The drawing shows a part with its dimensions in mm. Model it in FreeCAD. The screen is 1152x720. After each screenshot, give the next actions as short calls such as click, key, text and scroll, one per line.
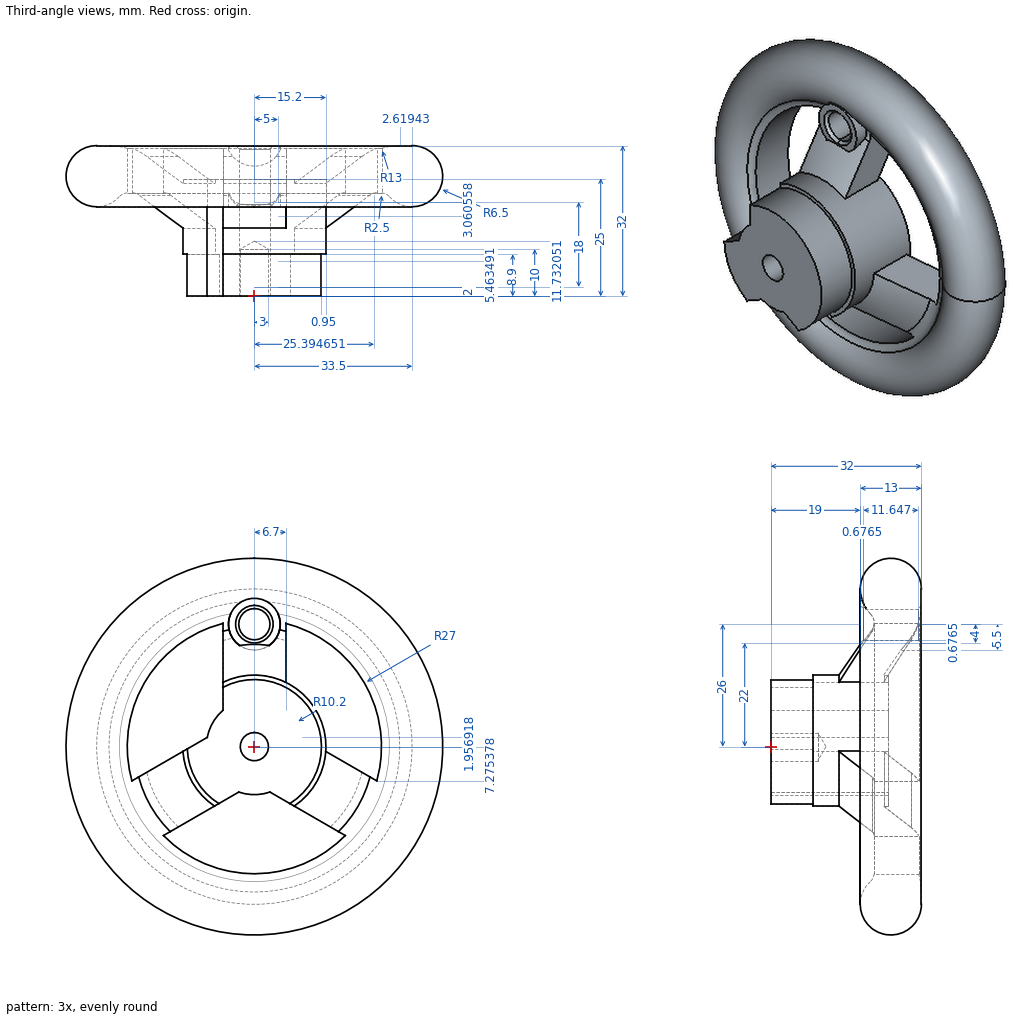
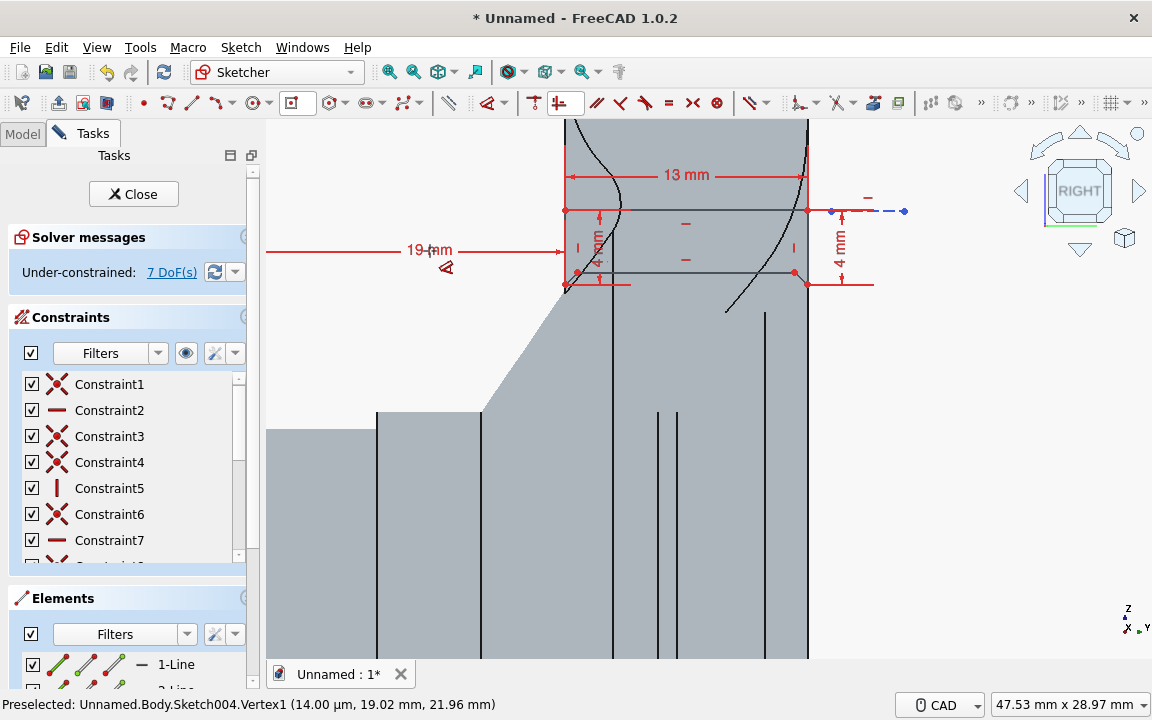
click(565, 285)
click(599, 458)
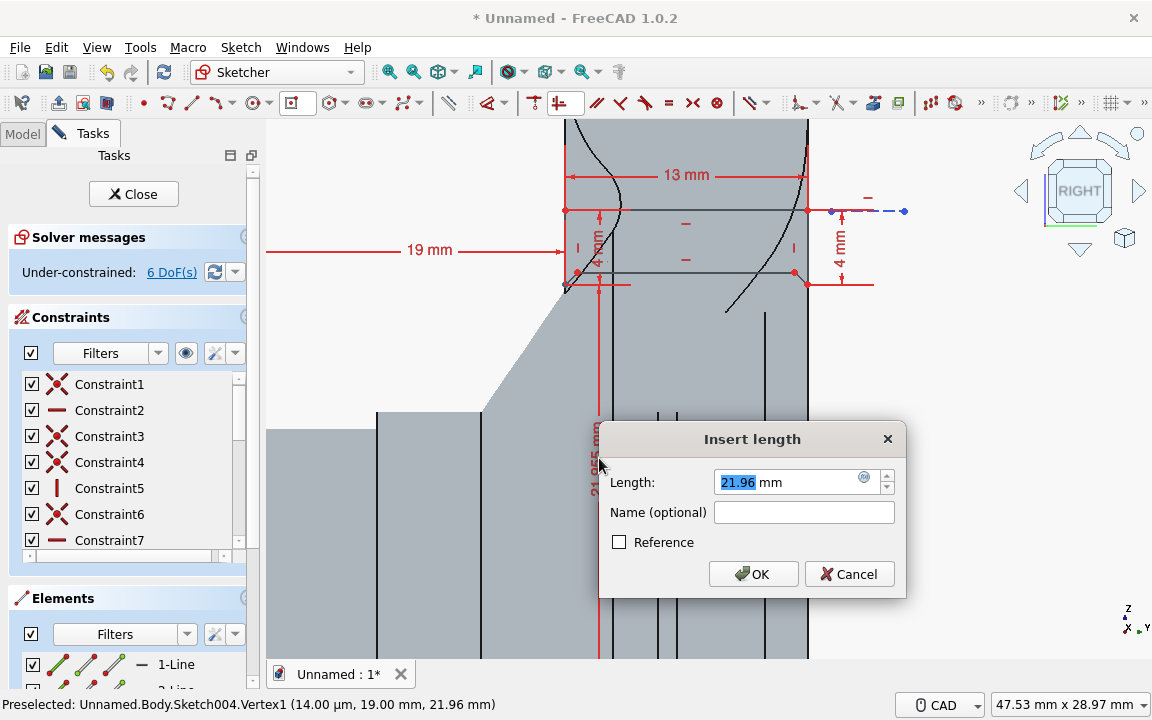
text(22)
key(Return)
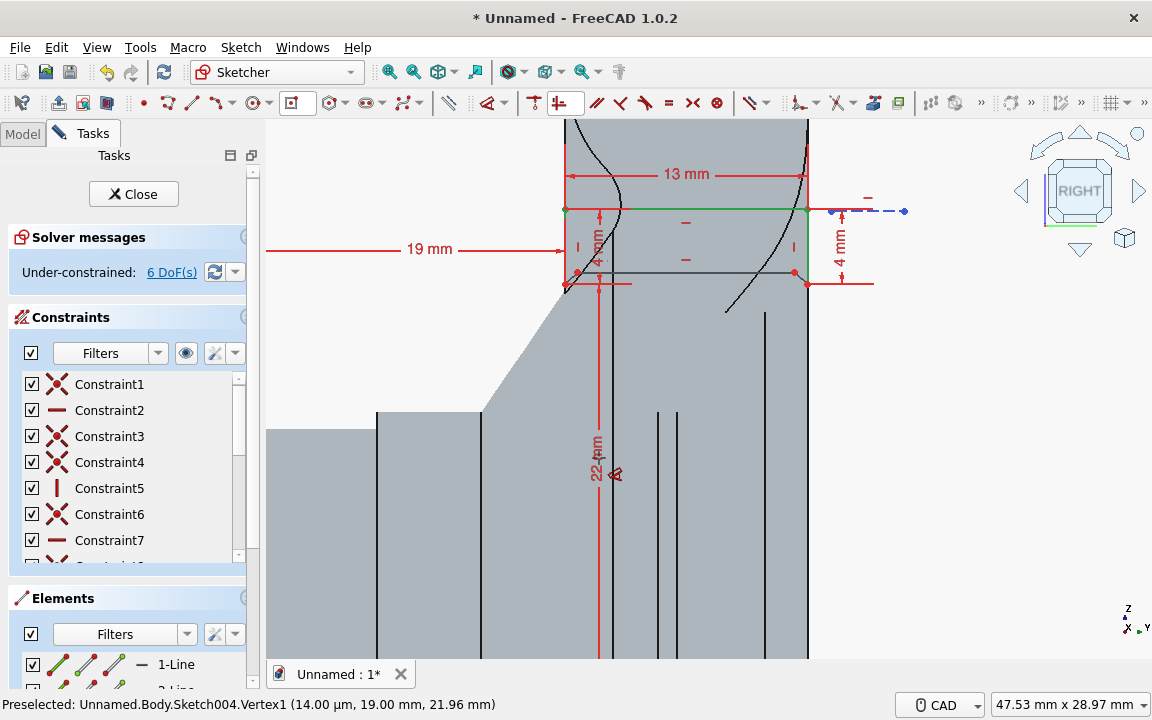
click(832, 211)
click(866, 421)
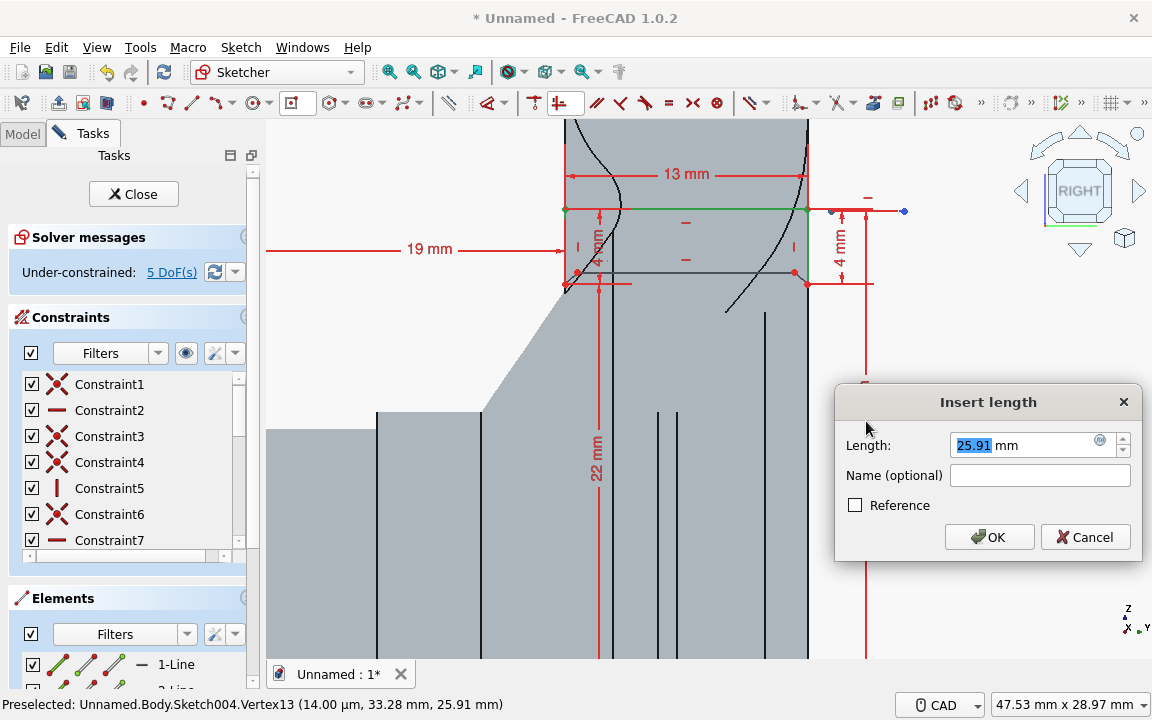
text(26)
key(Return)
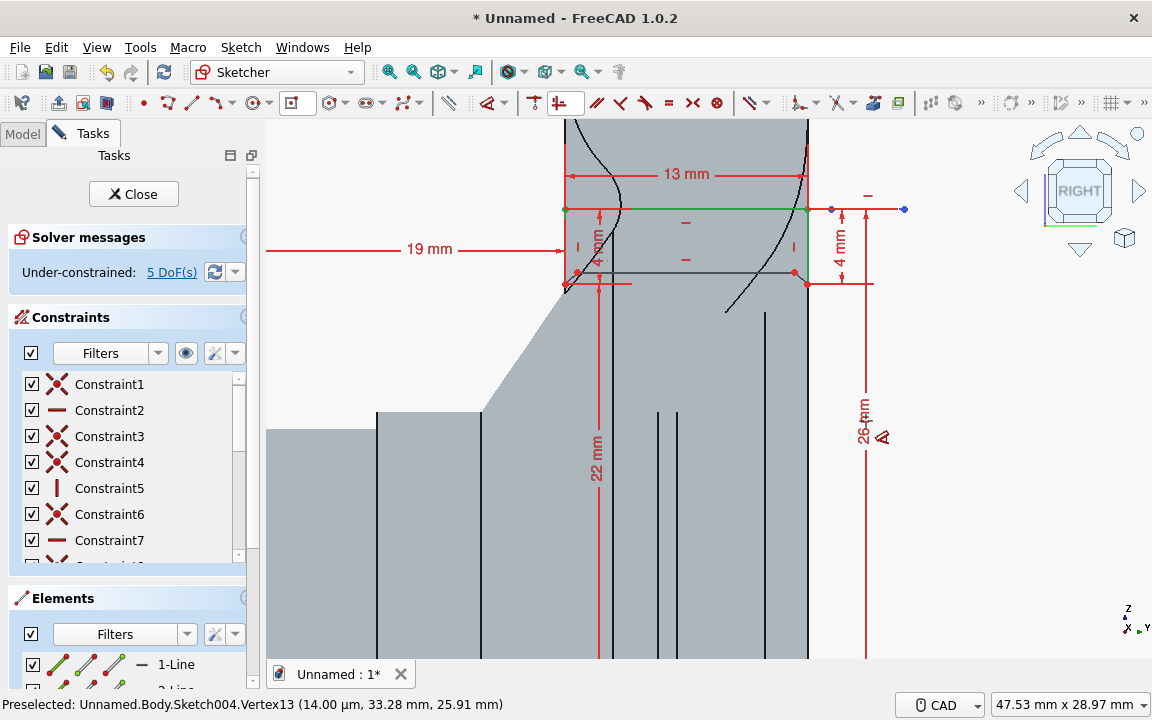
click(643, 273)
click(686, 239)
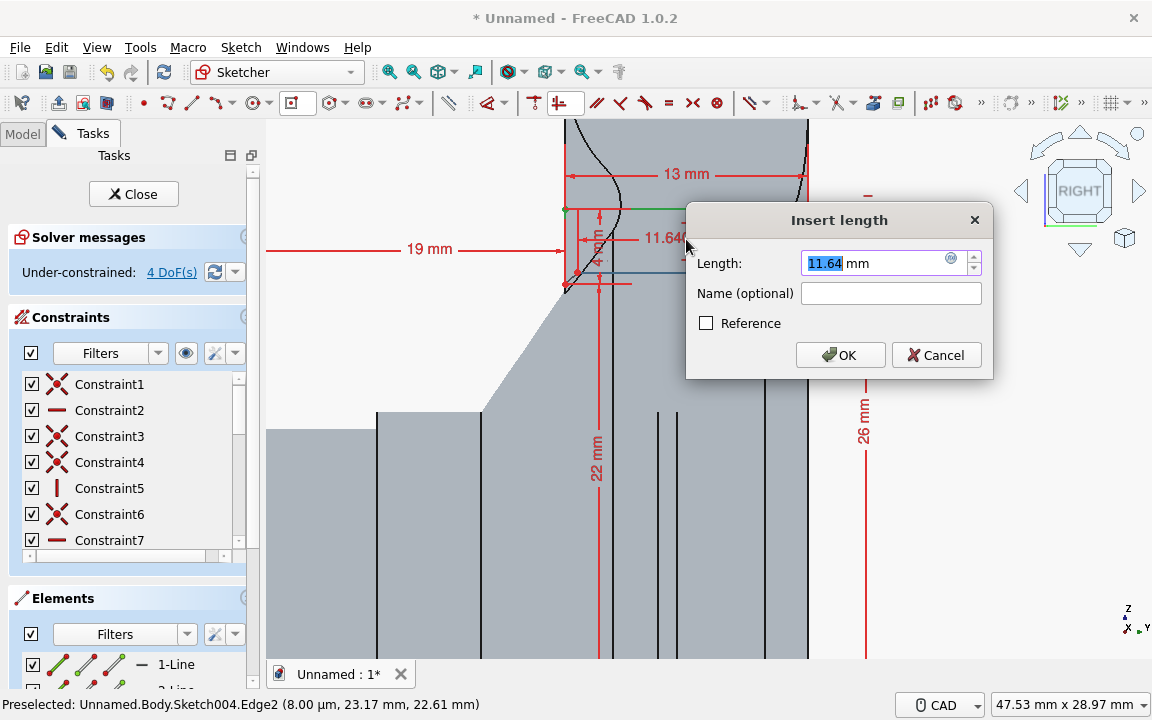
text(11.647)
key(Return)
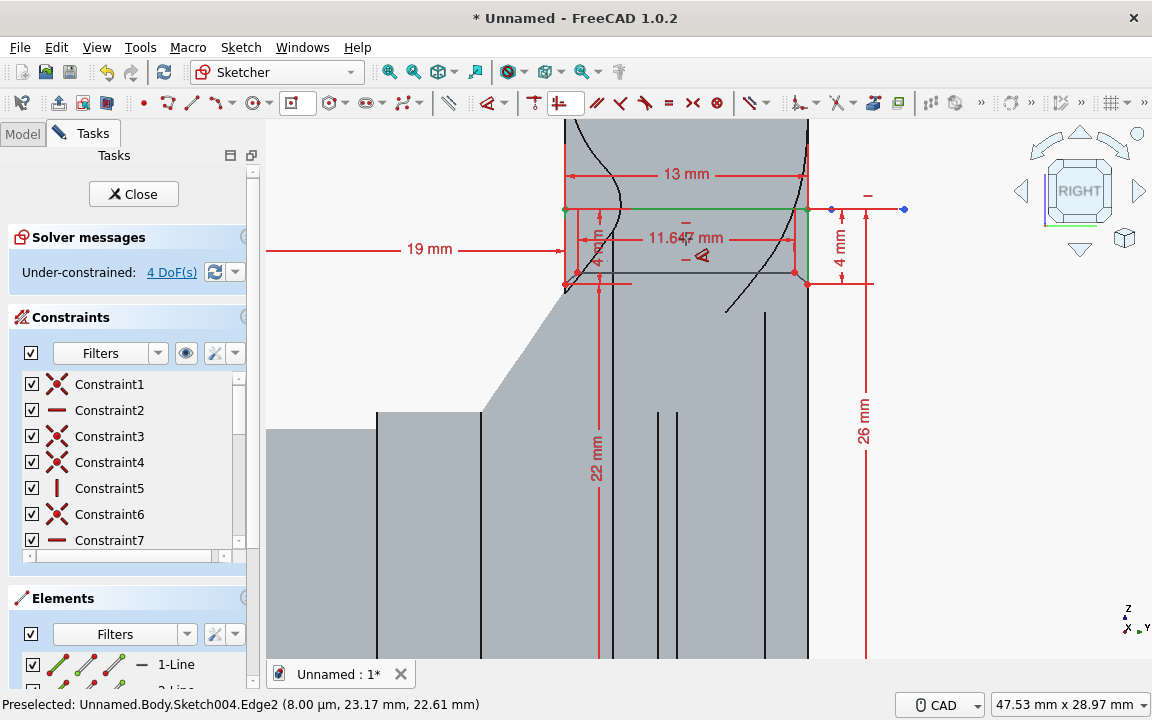
scroll(573, 277, up, 6)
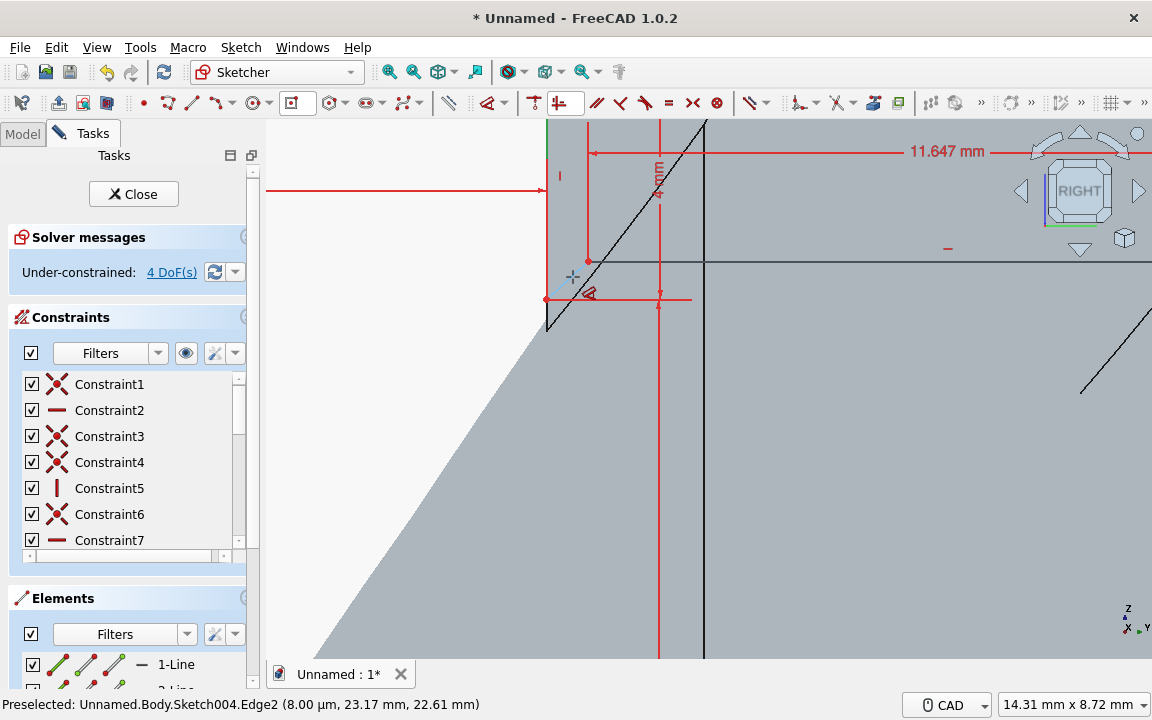
click(572, 277)
click(567, 228)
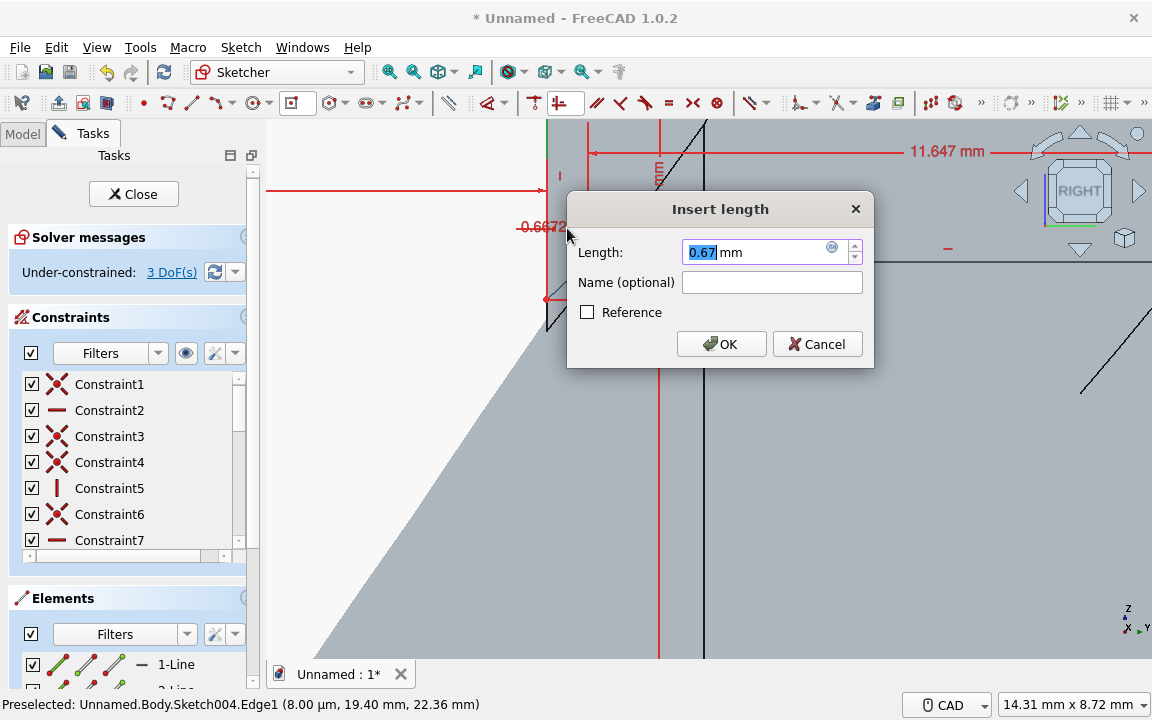
text(0.6765)
key(Return)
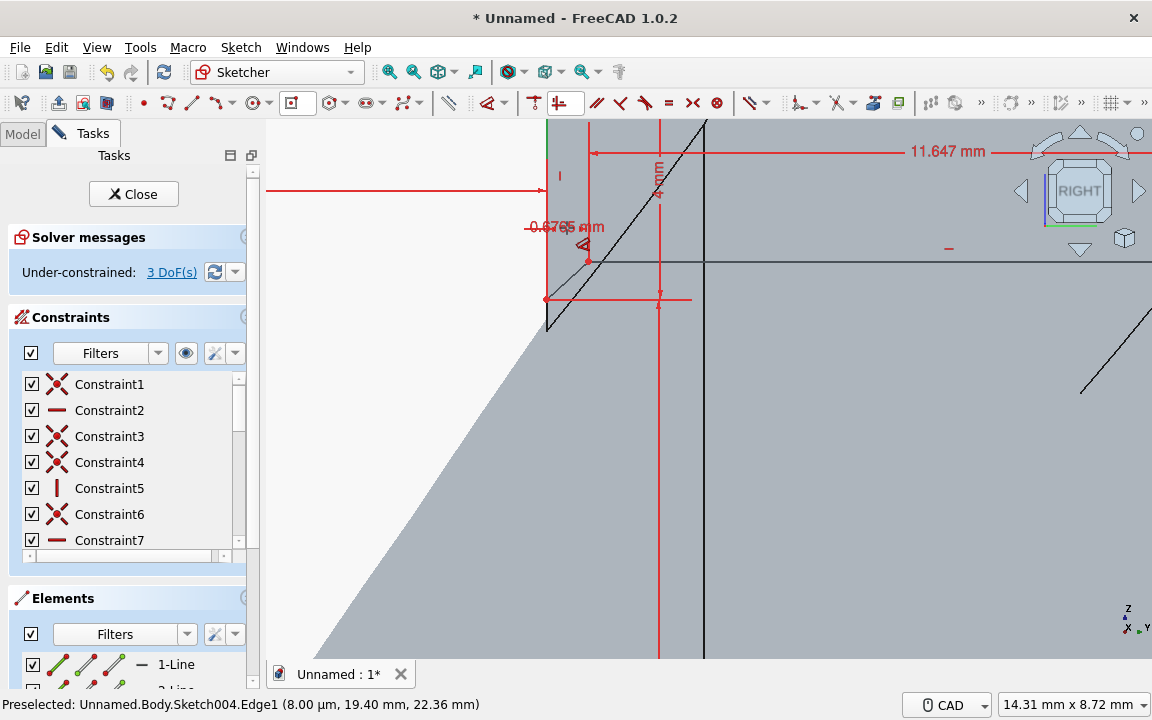
click(559, 288)
click(623, 281)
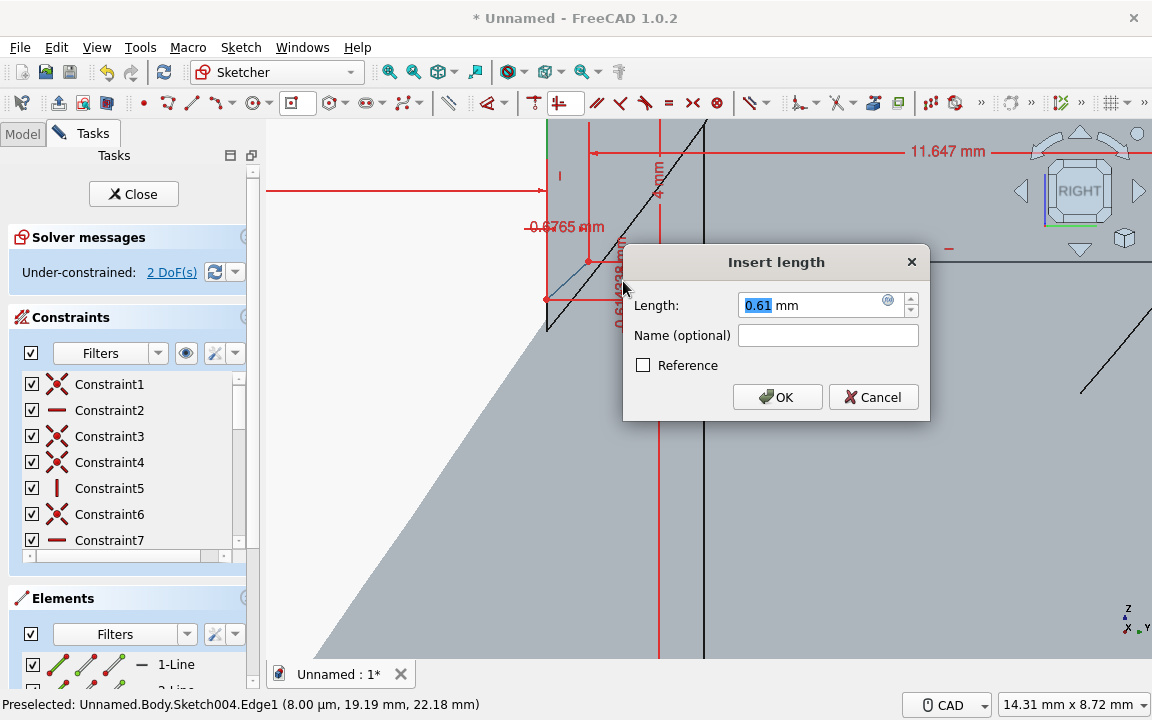
text(0.6765)
key(Return)
key(Escape)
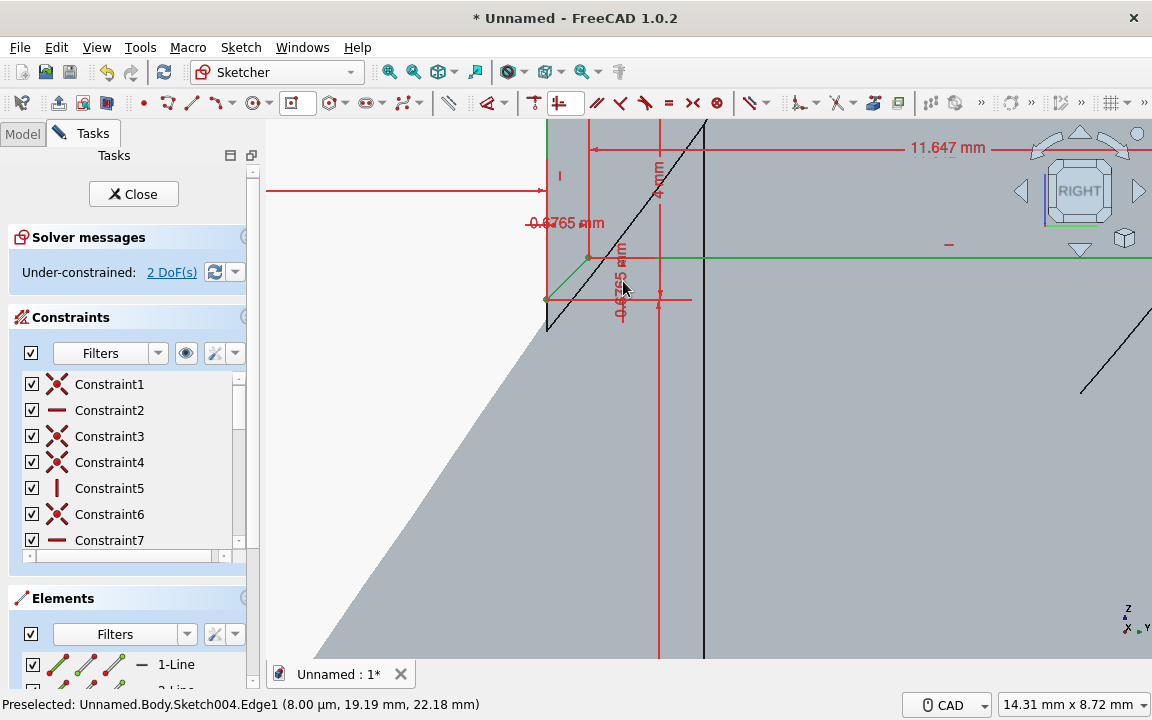
click(134, 194)